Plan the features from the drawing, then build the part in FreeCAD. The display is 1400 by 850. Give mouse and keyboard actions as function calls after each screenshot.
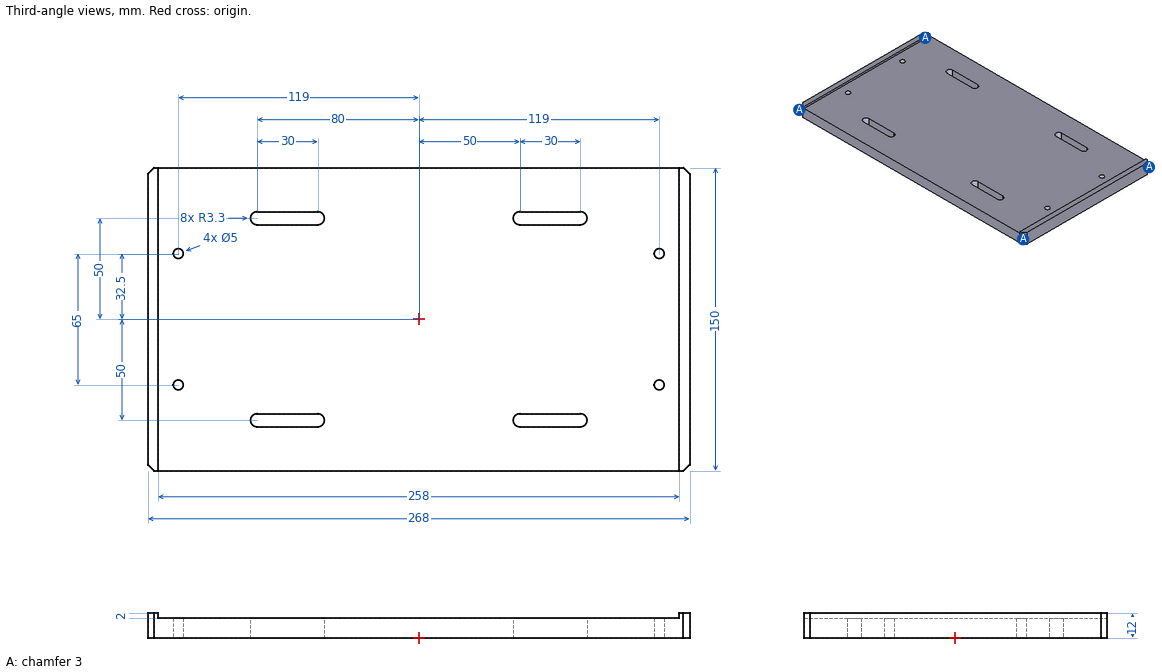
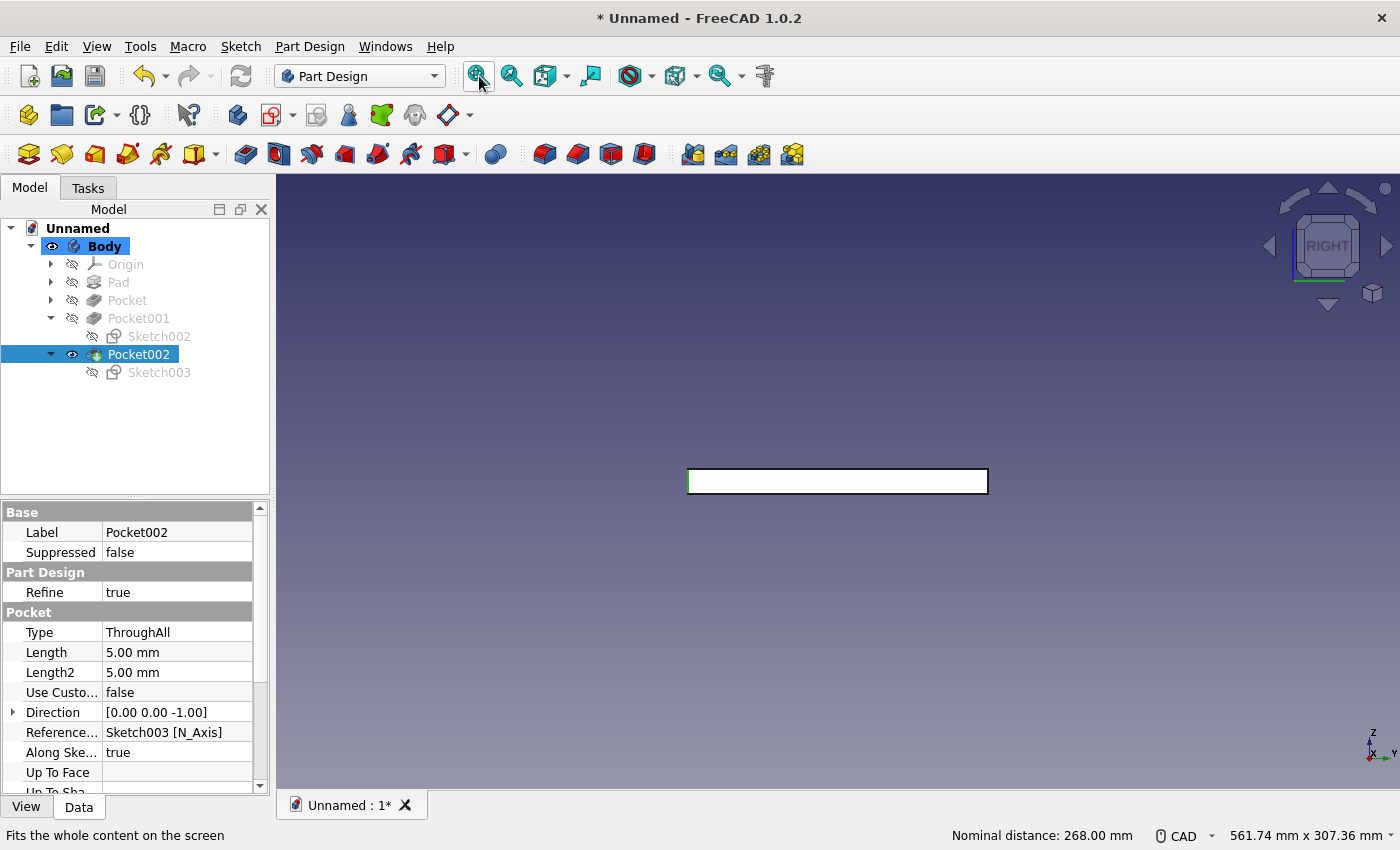
click(988, 480, ctrl)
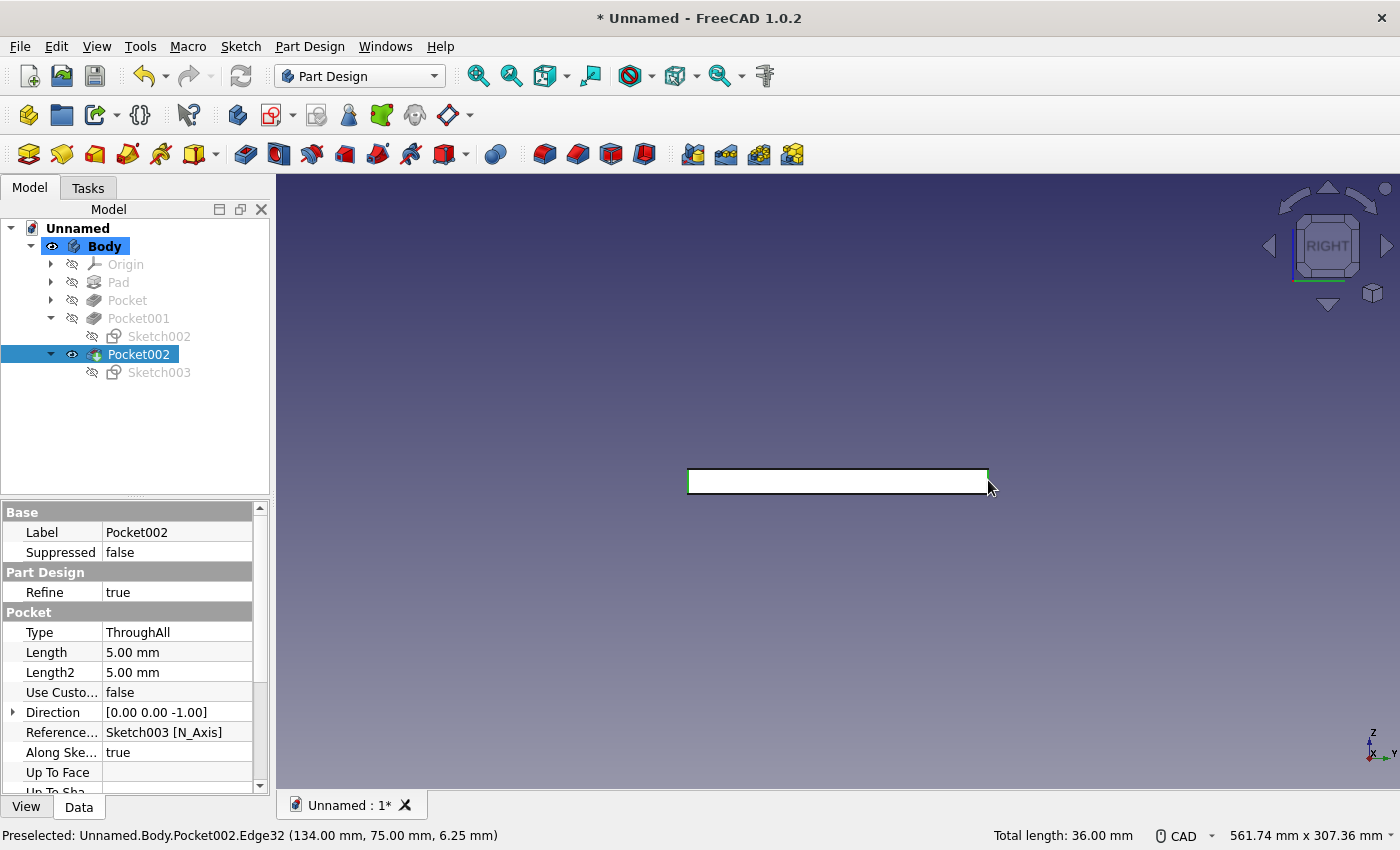
key(5)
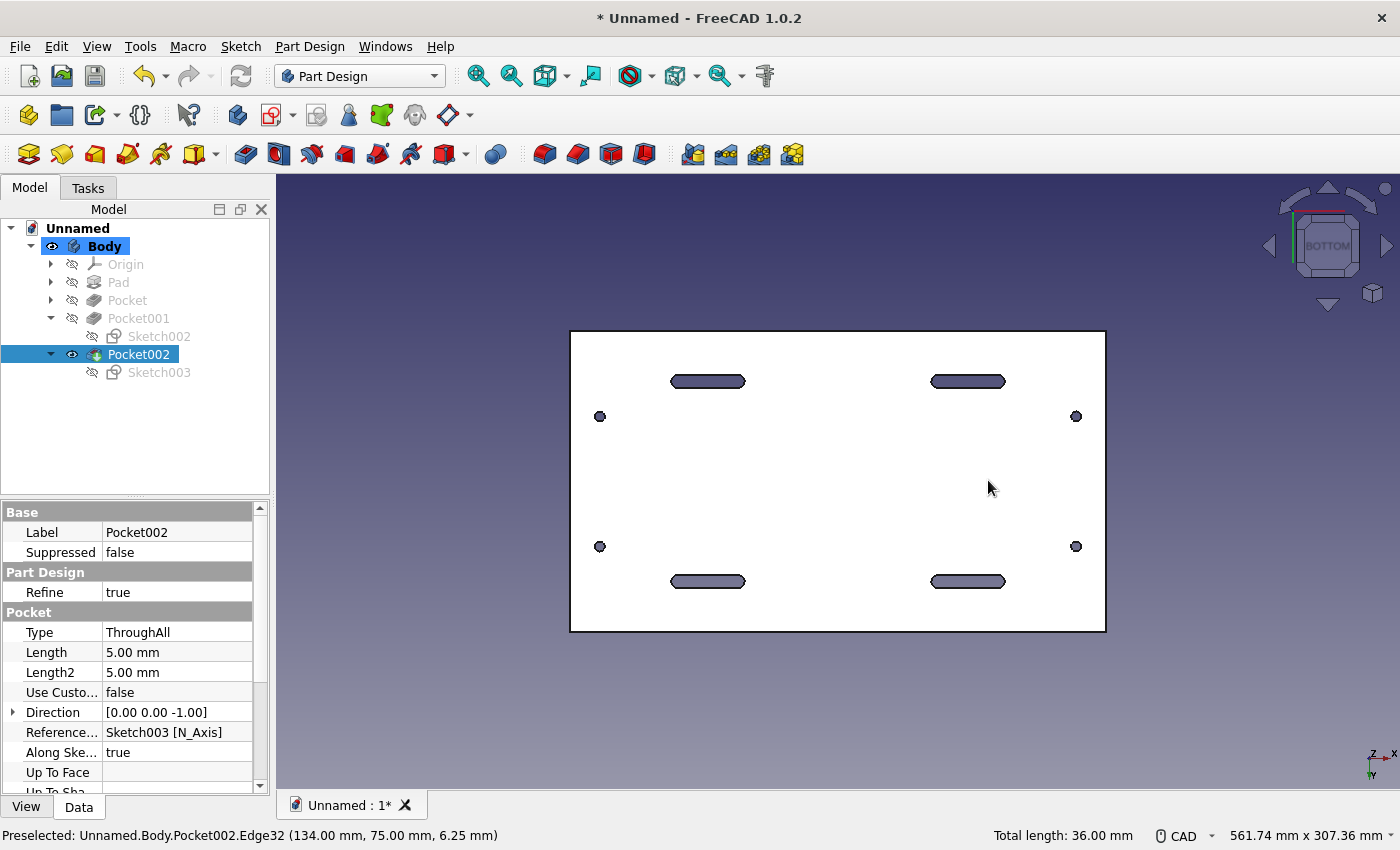
key(4)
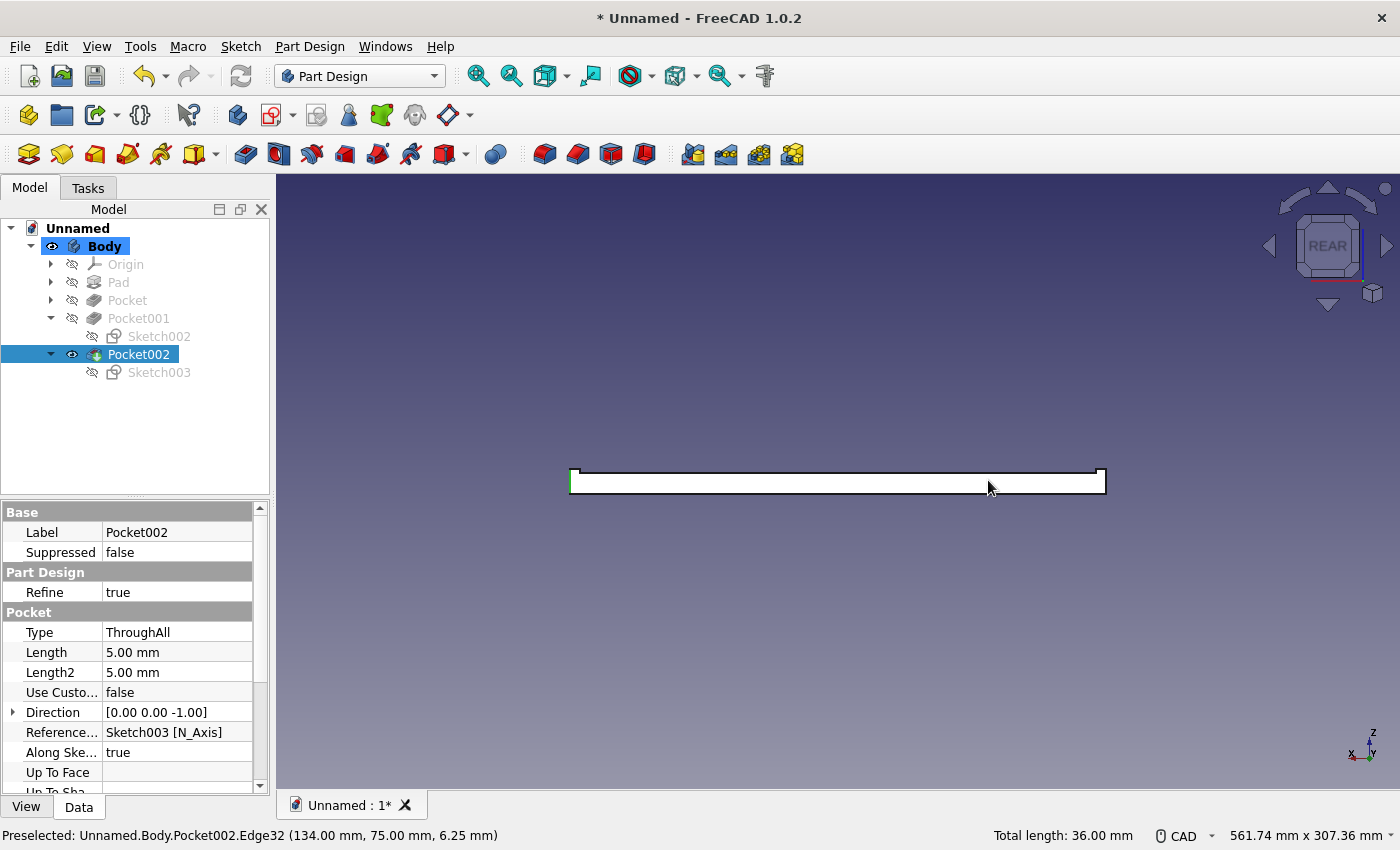
click(1106, 480, ctrl)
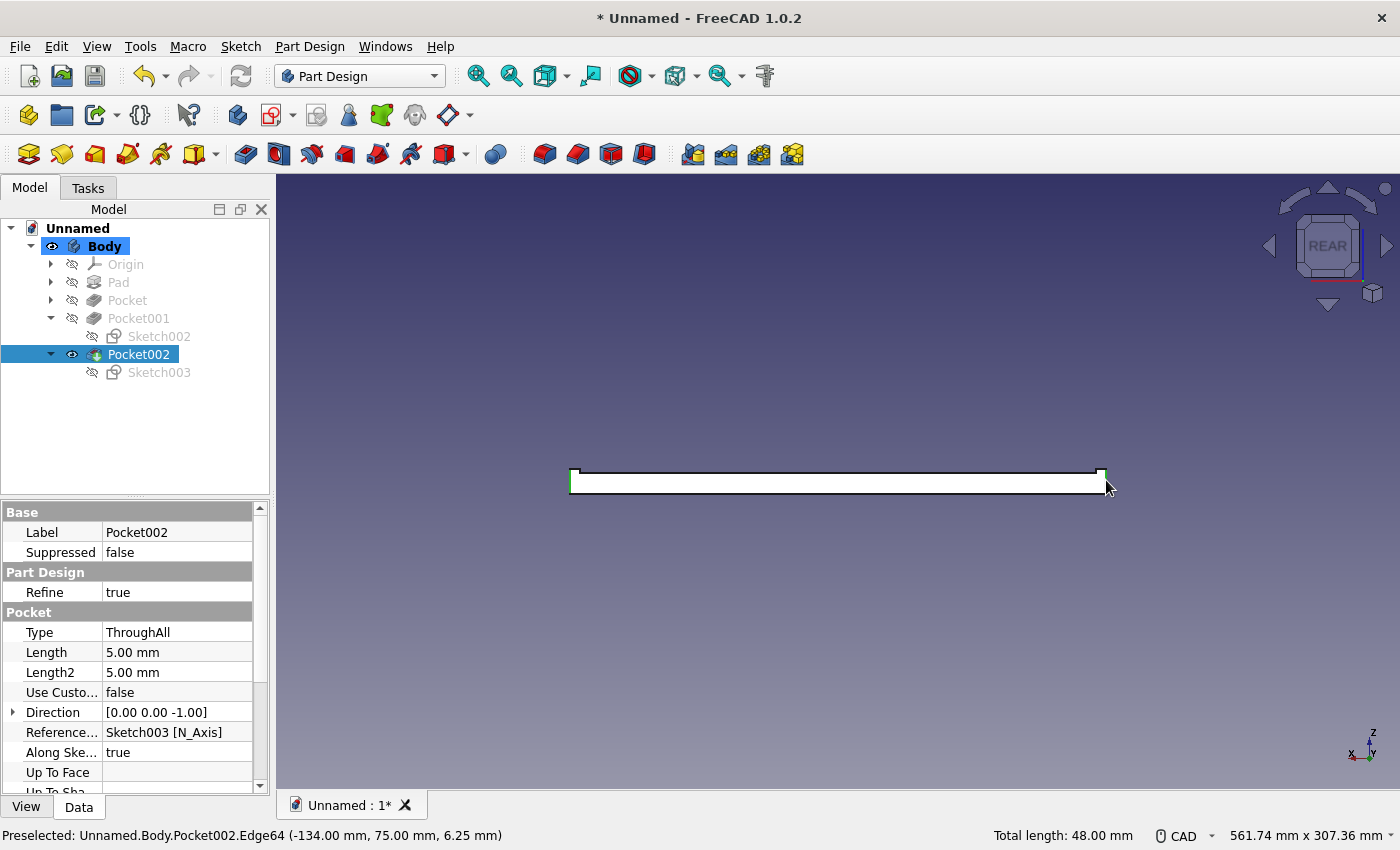
click(578, 154)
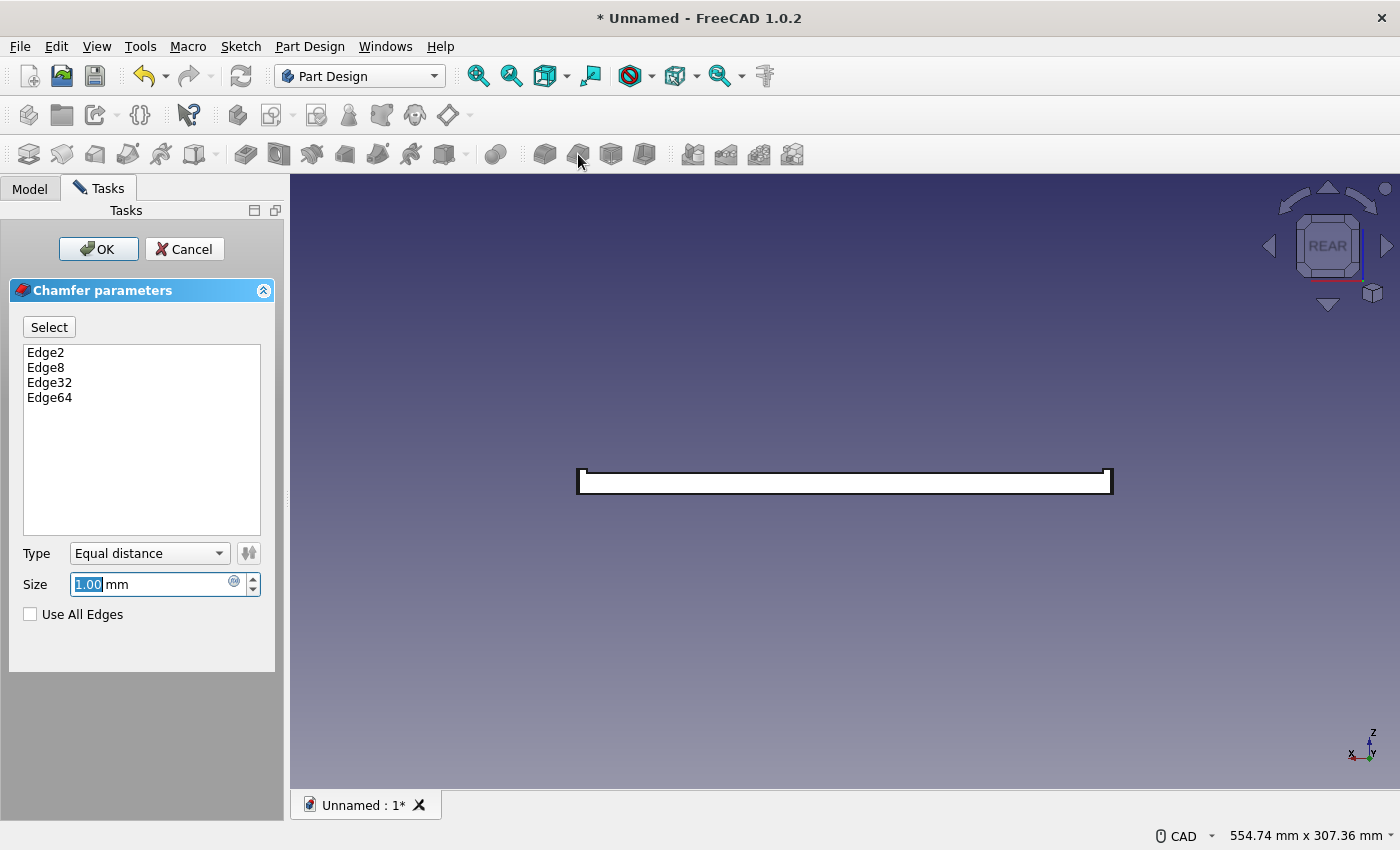
text(3)
key(Tab)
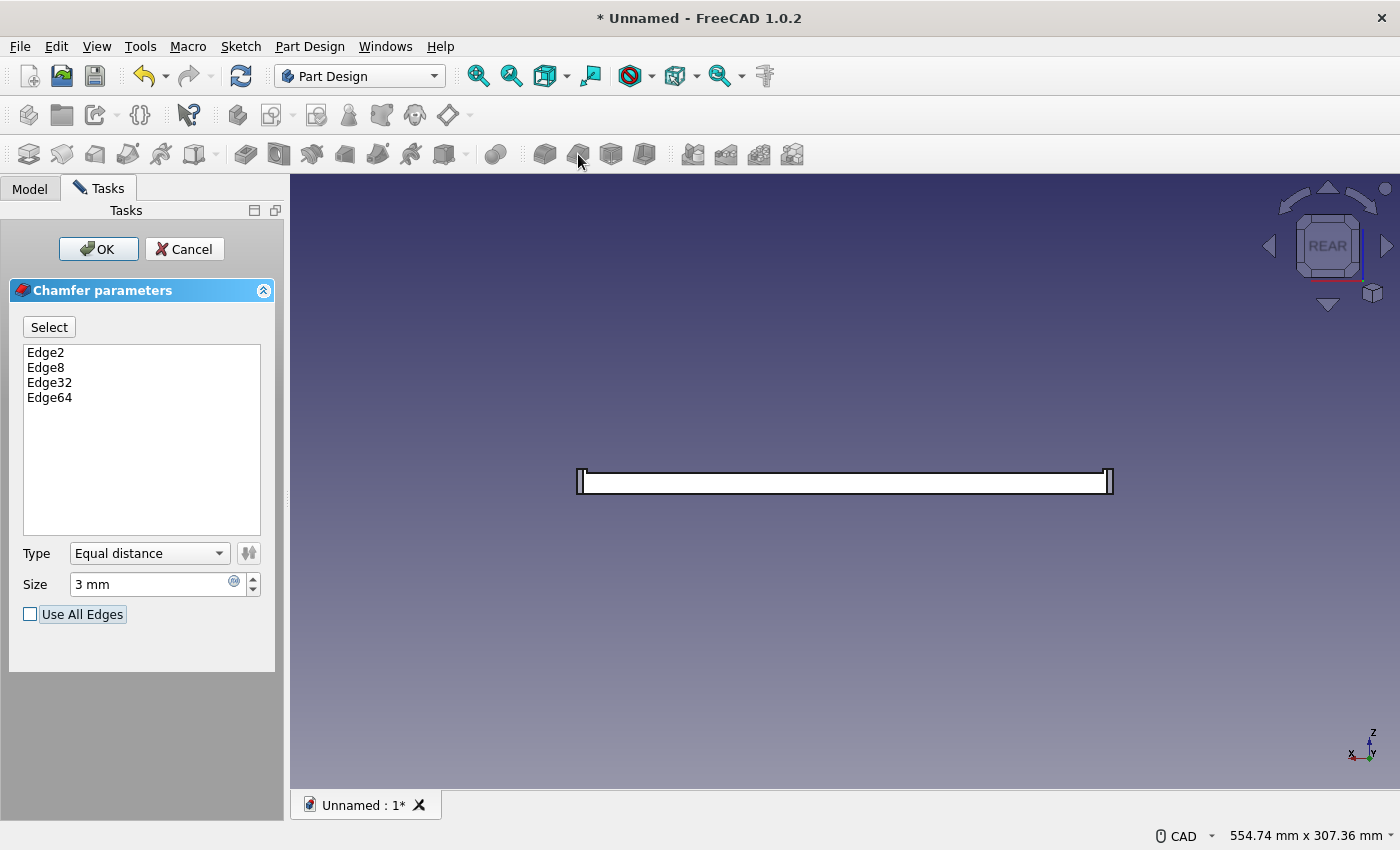
click(99, 249)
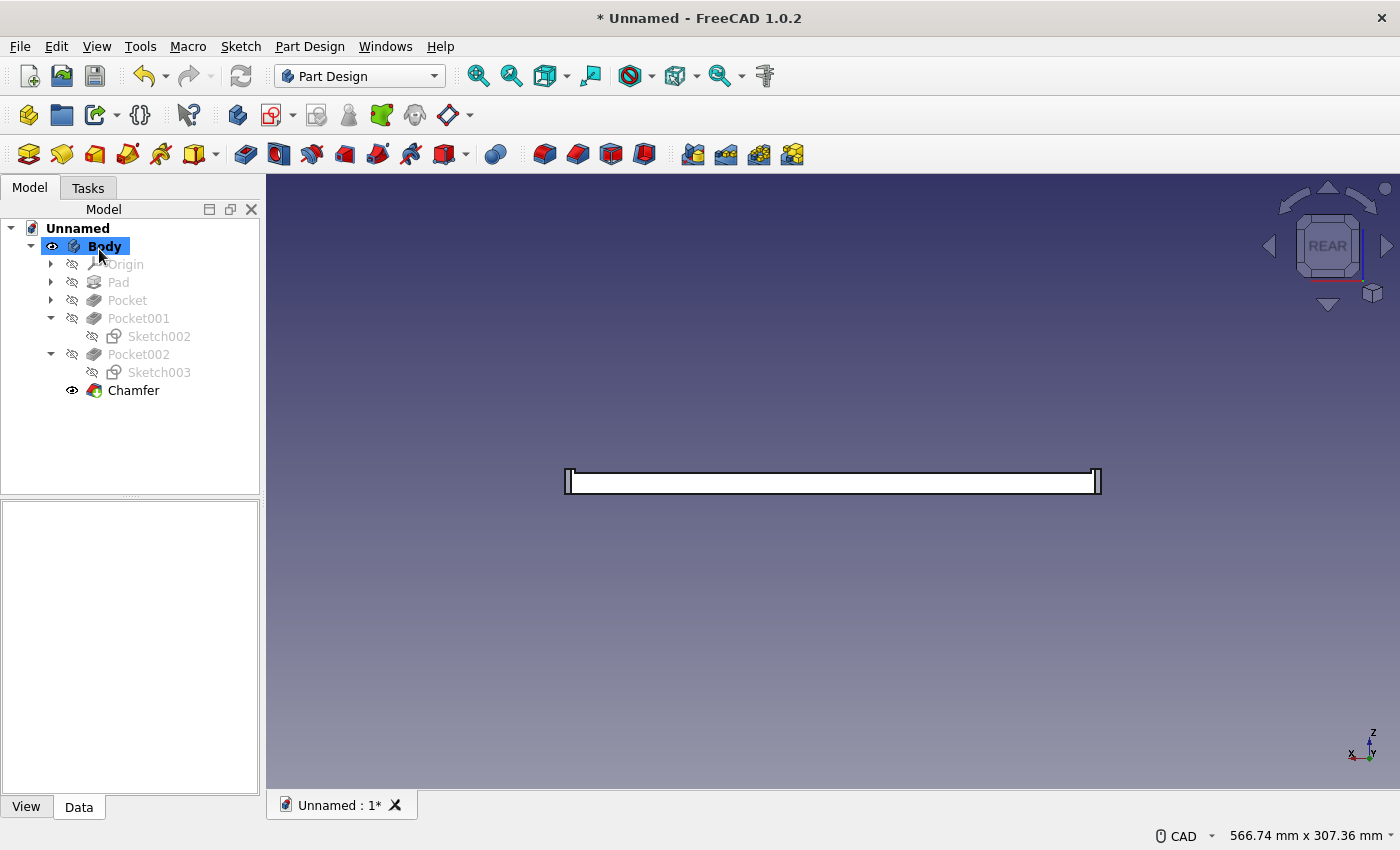
key(0)